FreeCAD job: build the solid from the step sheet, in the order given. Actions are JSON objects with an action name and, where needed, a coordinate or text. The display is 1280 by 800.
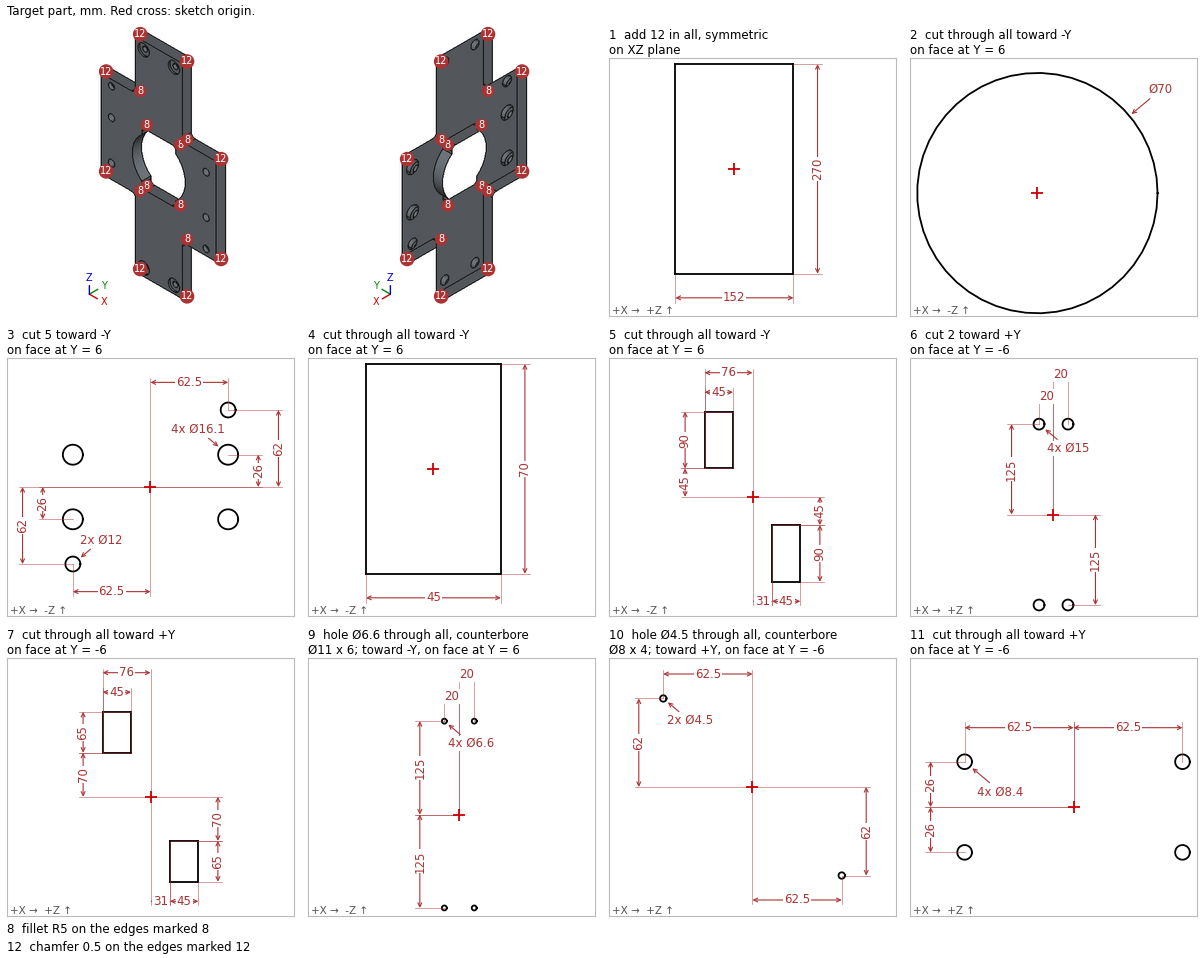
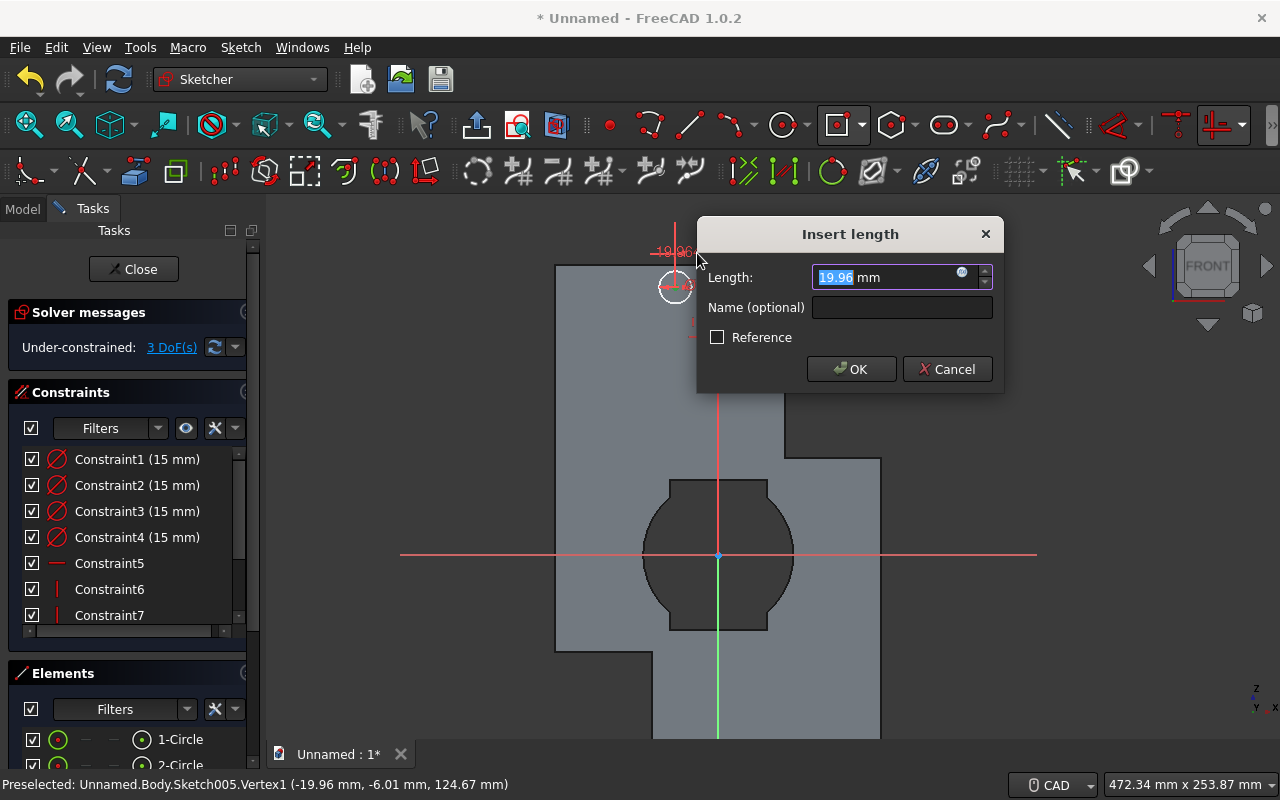
{"action": "type", "text": "20"}
{"action": "key", "text": "Return"}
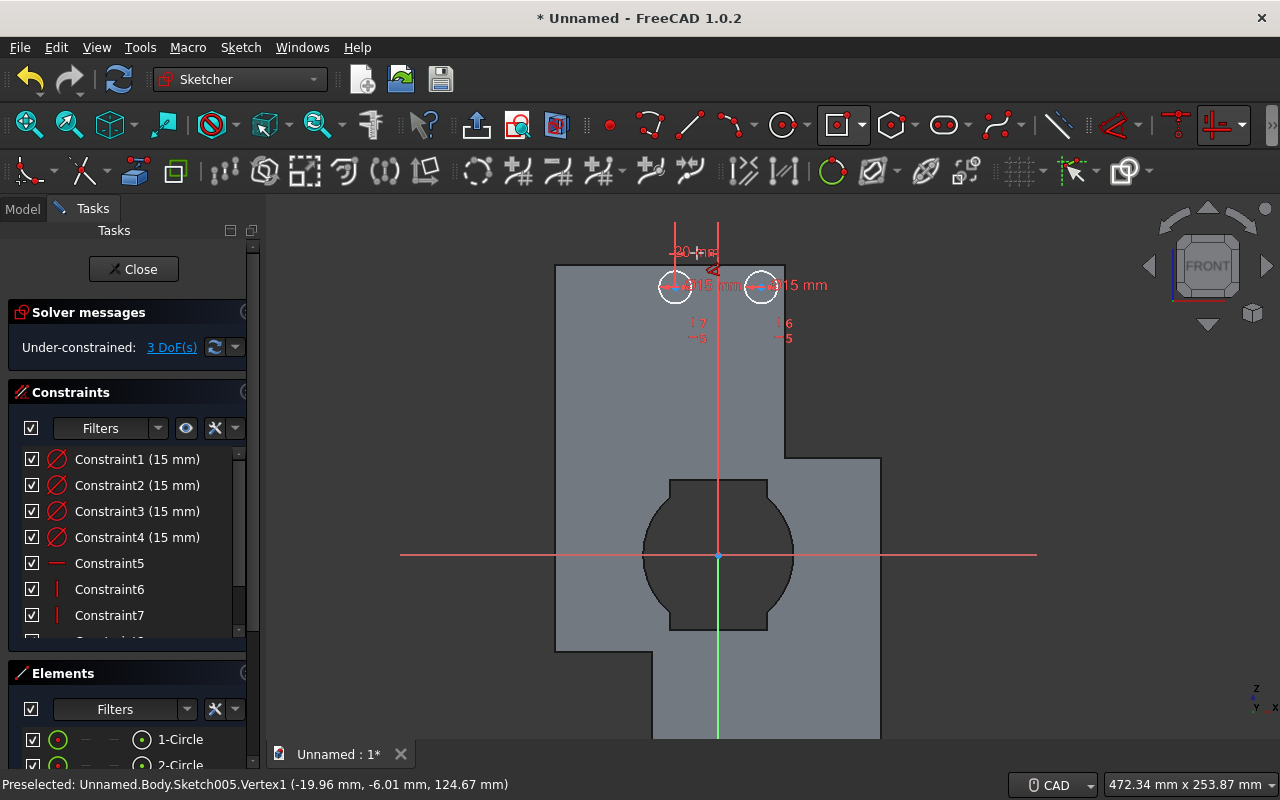
{"action": "left_click", "coordinate": [761, 287]}
{"action": "left_click", "coordinate": [740, 589]}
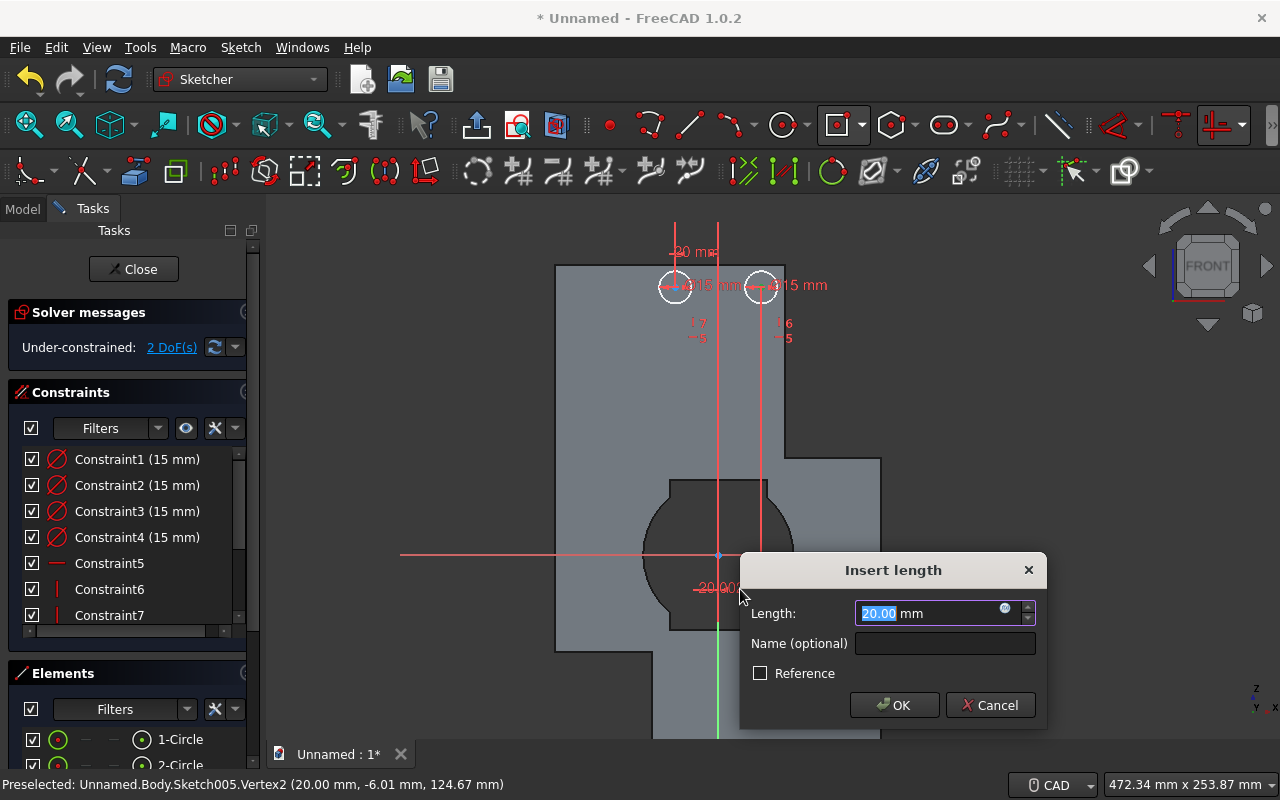
{"action": "type", "text": "20"}
{"action": "key", "text": "Return"}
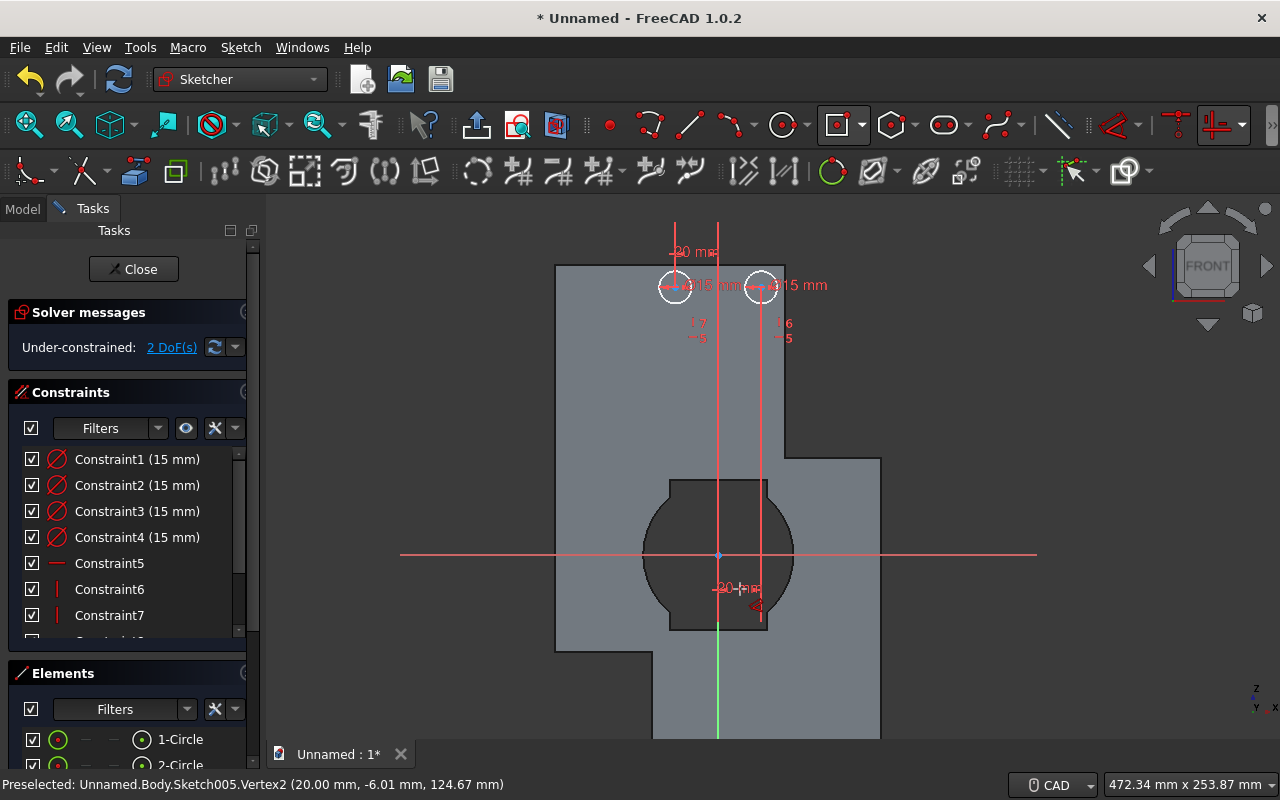
{"action": "left_click", "coordinate": [675, 287]}
{"action": "left_click", "coordinate": [641, 421]}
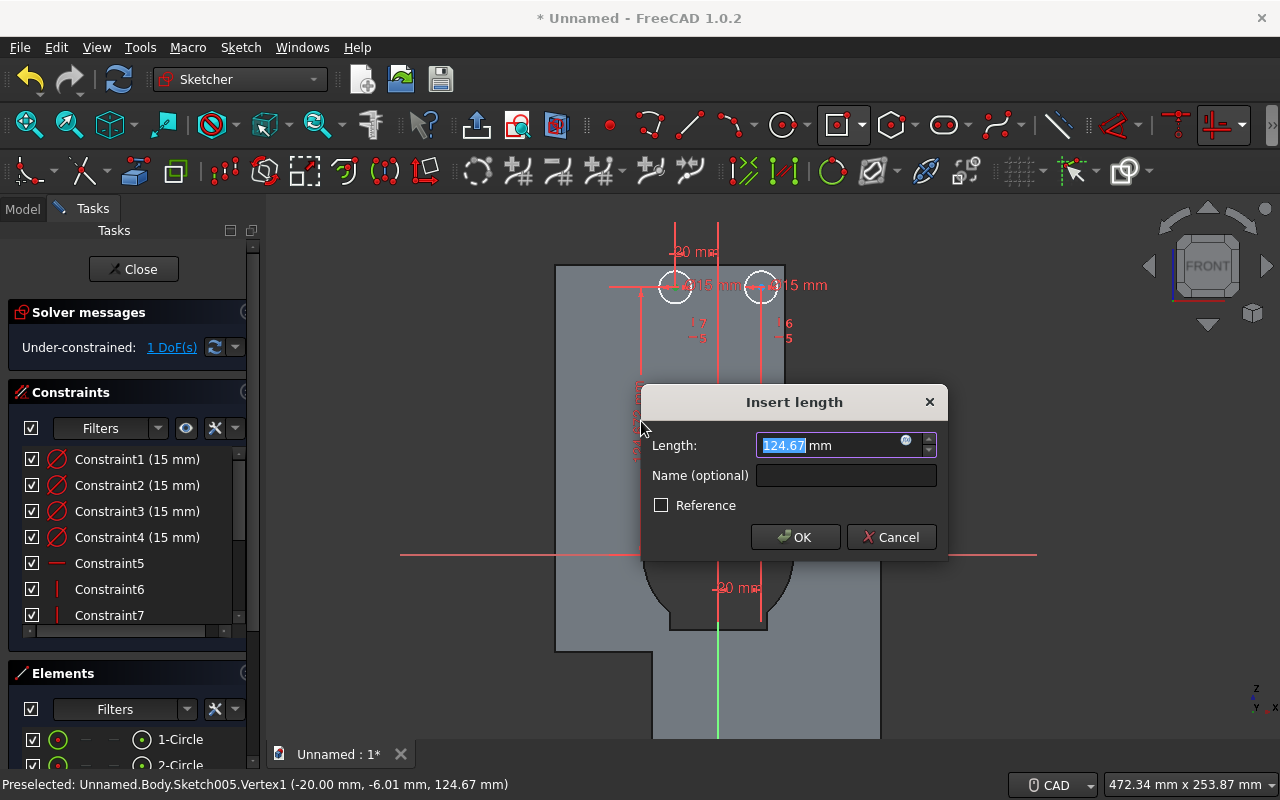
{"action": "type", "text": "125"}
{"action": "key", "text": "Return"}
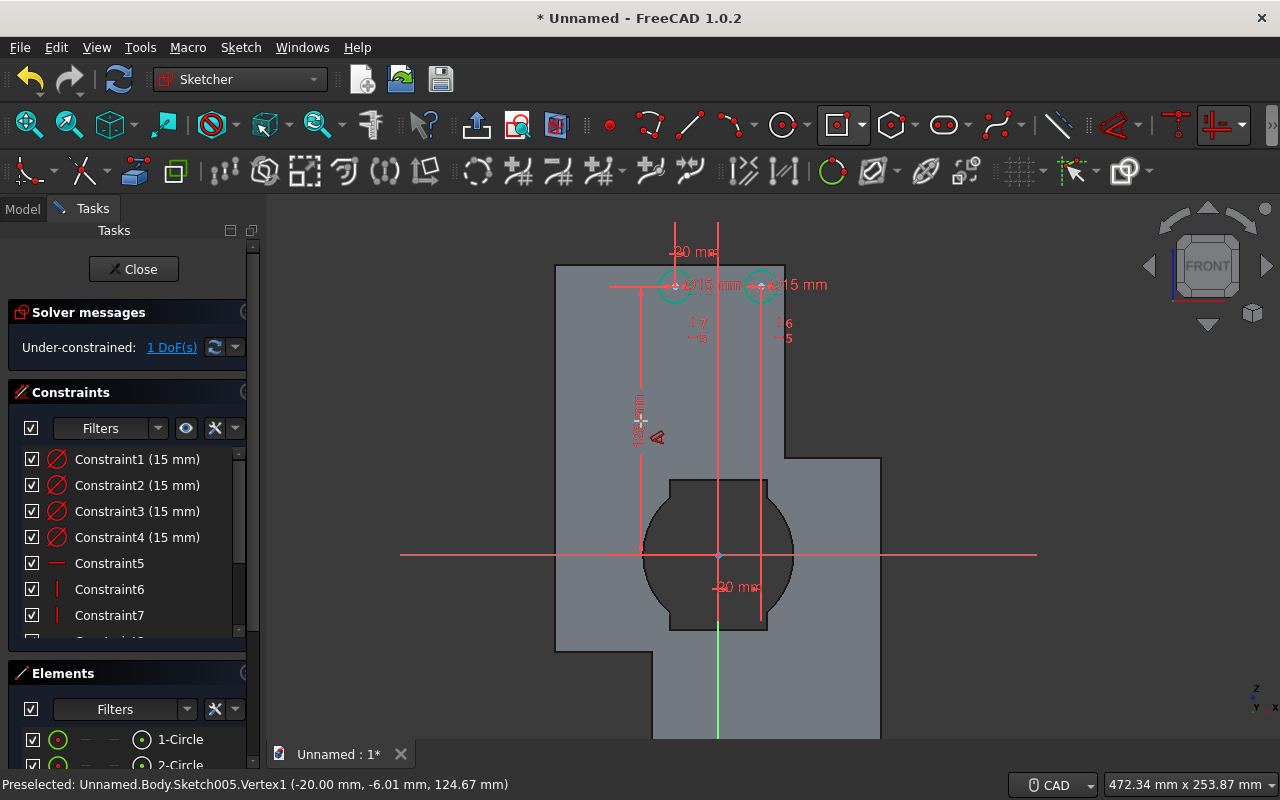
{"action": "scroll", "coordinate": [676, 286], "scroll_direction": "down", "scroll_amount": 2}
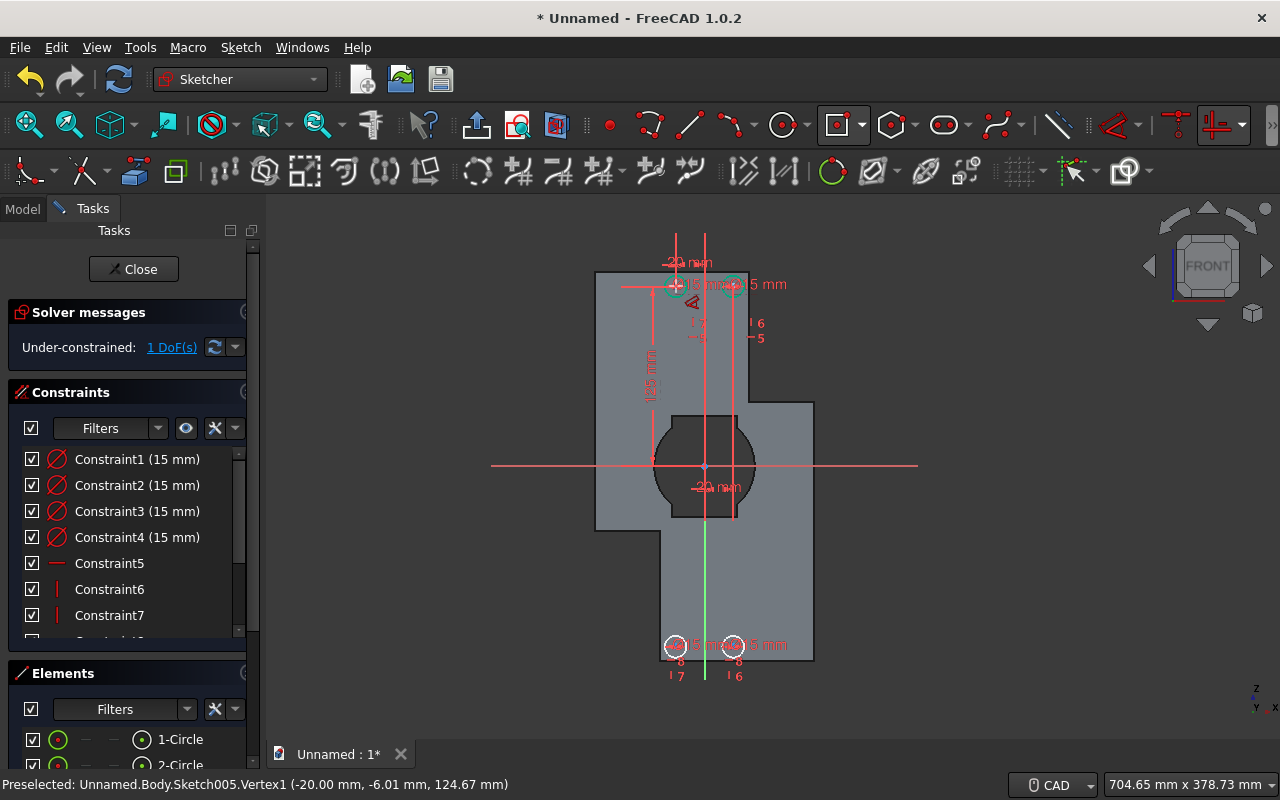
{"action": "left_click", "coordinate": [733, 647]}
{"action": "left_click", "coordinate": [767, 557]}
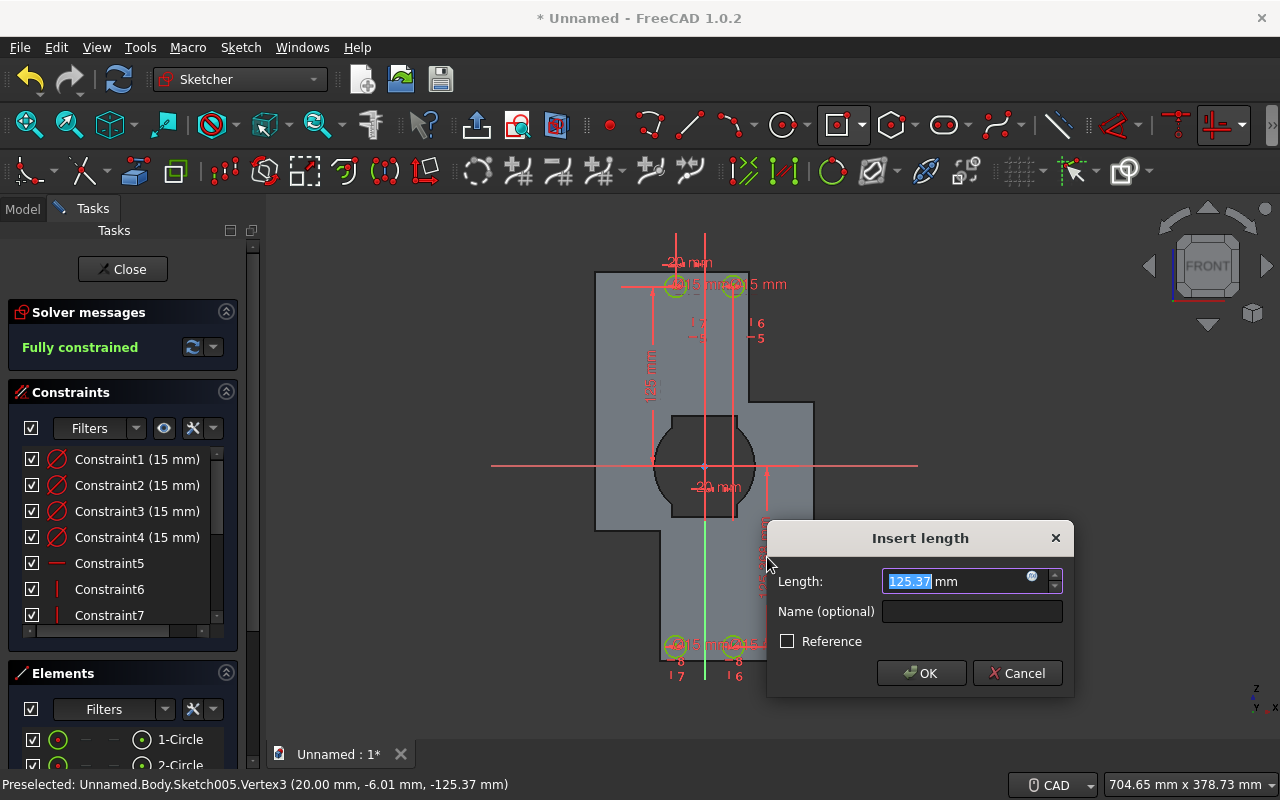
{"action": "type", "text": "125"}
{"action": "key", "text": "Return"}
{"action": "key", "text": "Escape"}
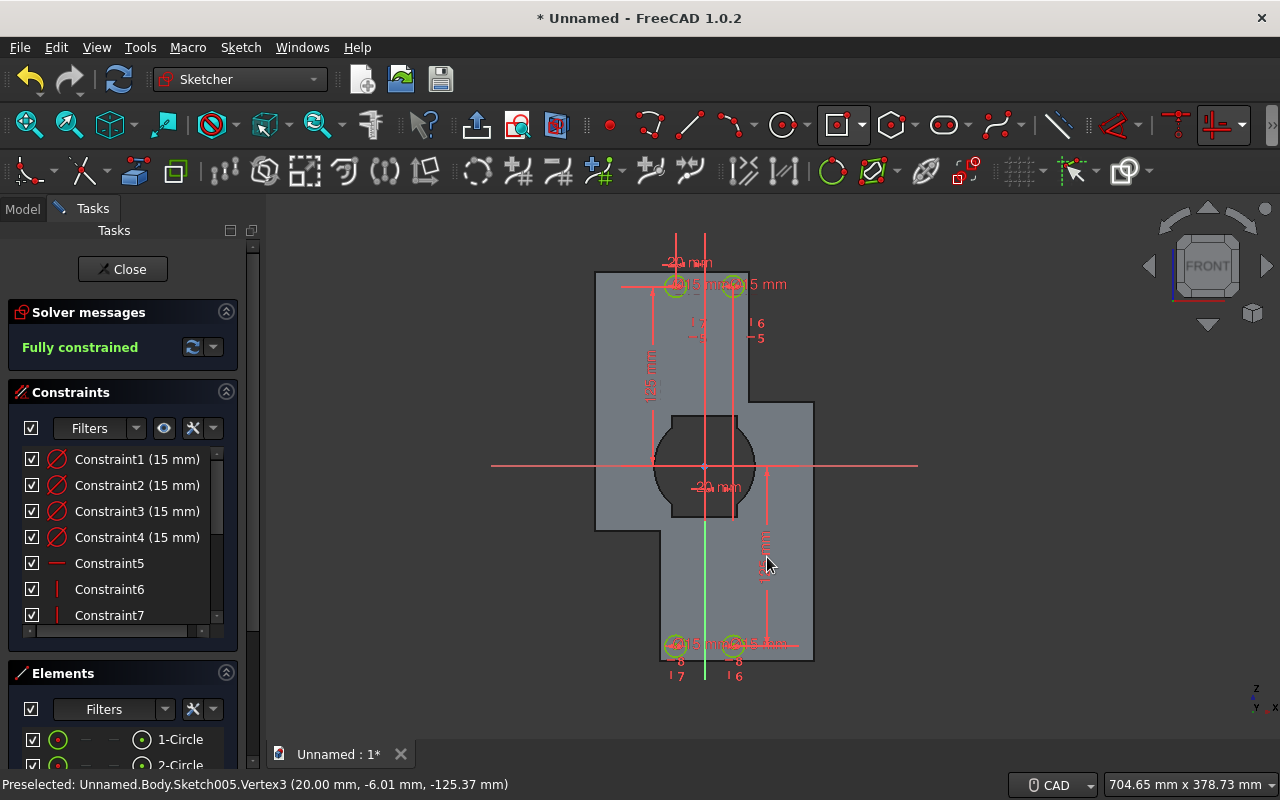
{"action": "left_click", "coordinate": [123, 269]}